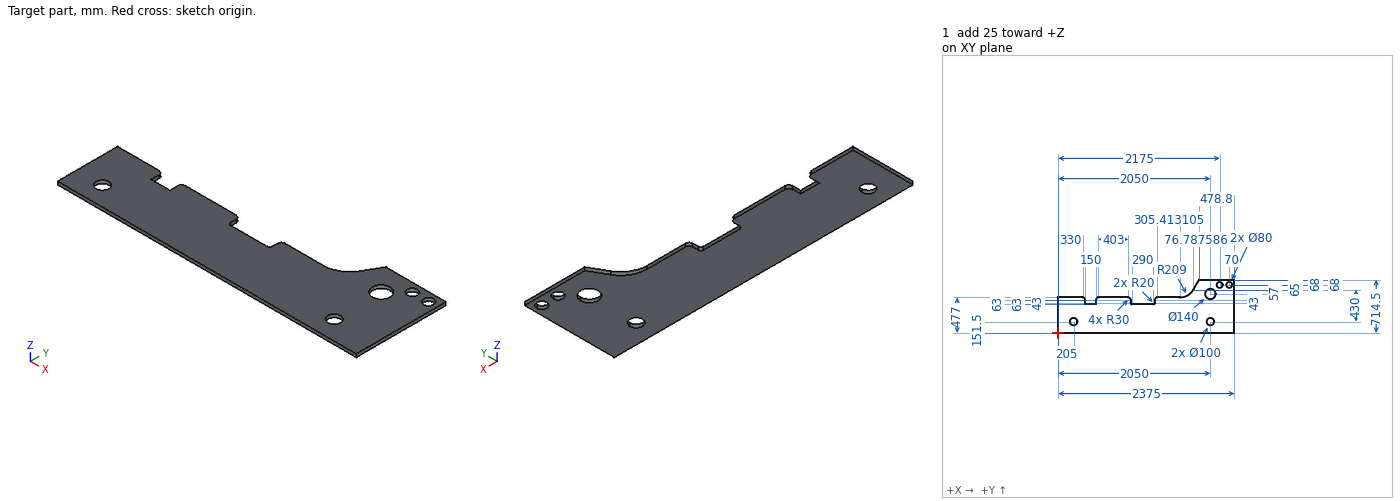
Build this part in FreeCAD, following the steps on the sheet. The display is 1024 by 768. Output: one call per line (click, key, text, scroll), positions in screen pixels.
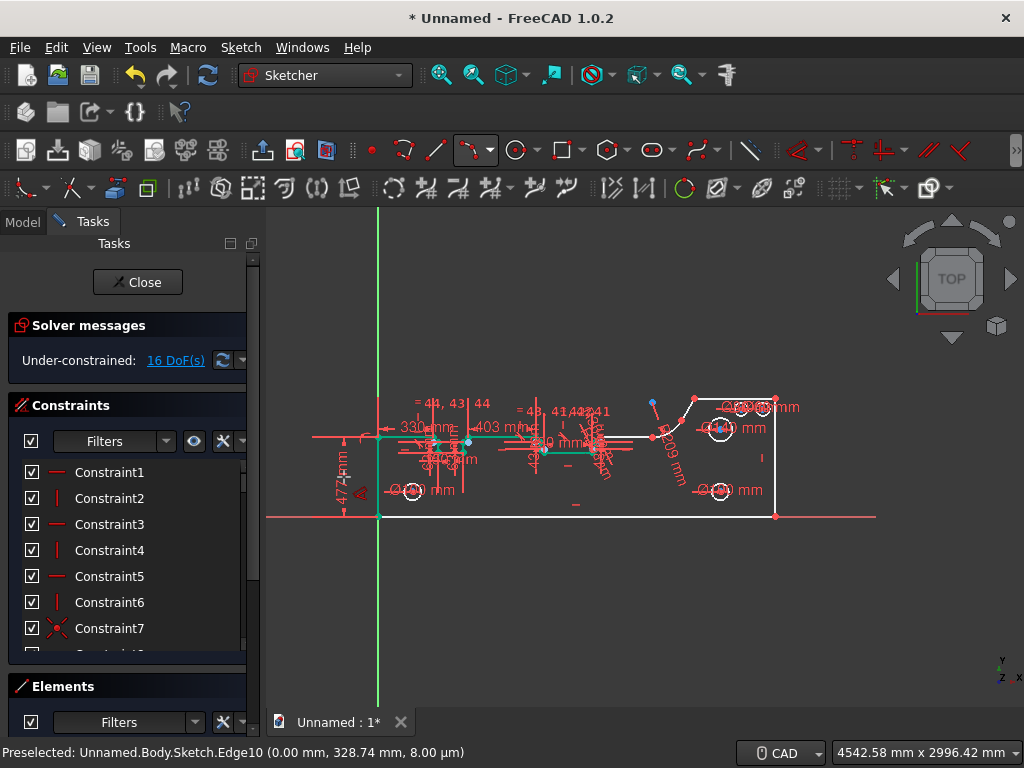
click(413, 492)
click(395, 551)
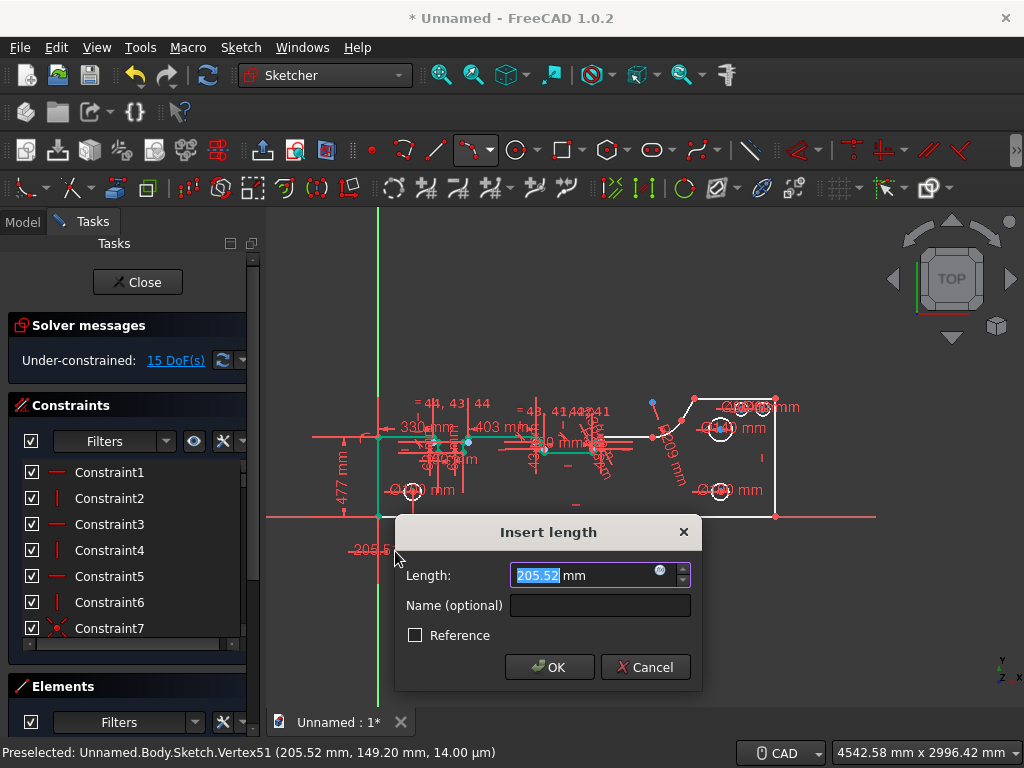
text(205)
key(Return)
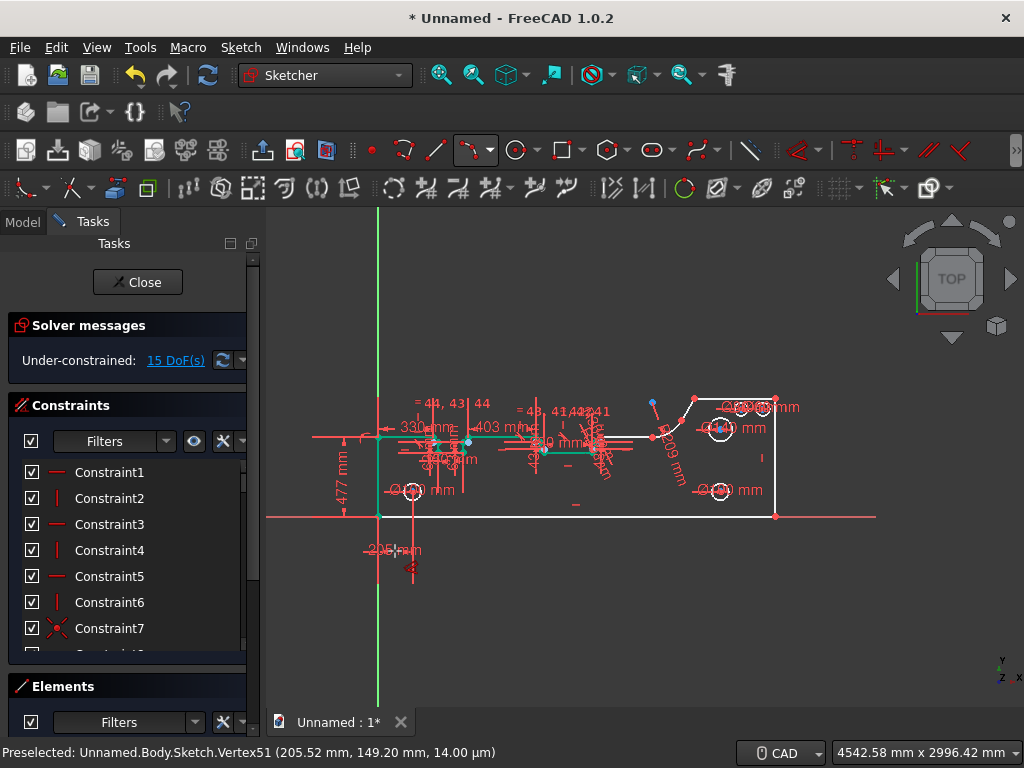
scroll(682, 421, up, 8)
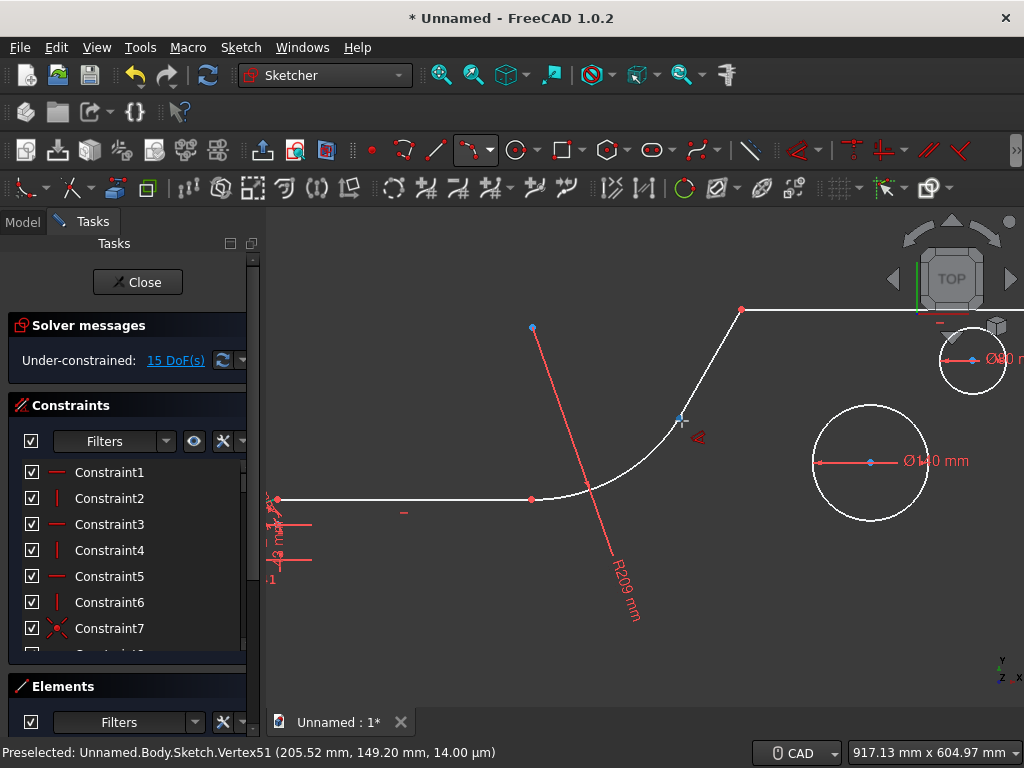
click(679, 418)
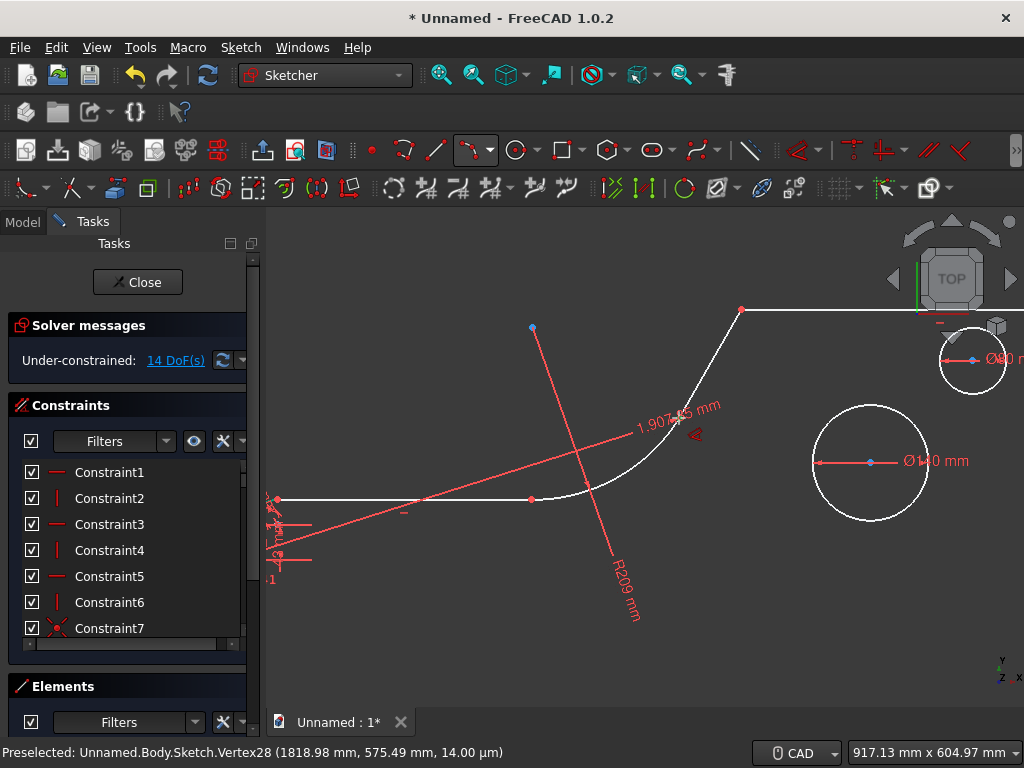
scroll(683, 421, down, 8)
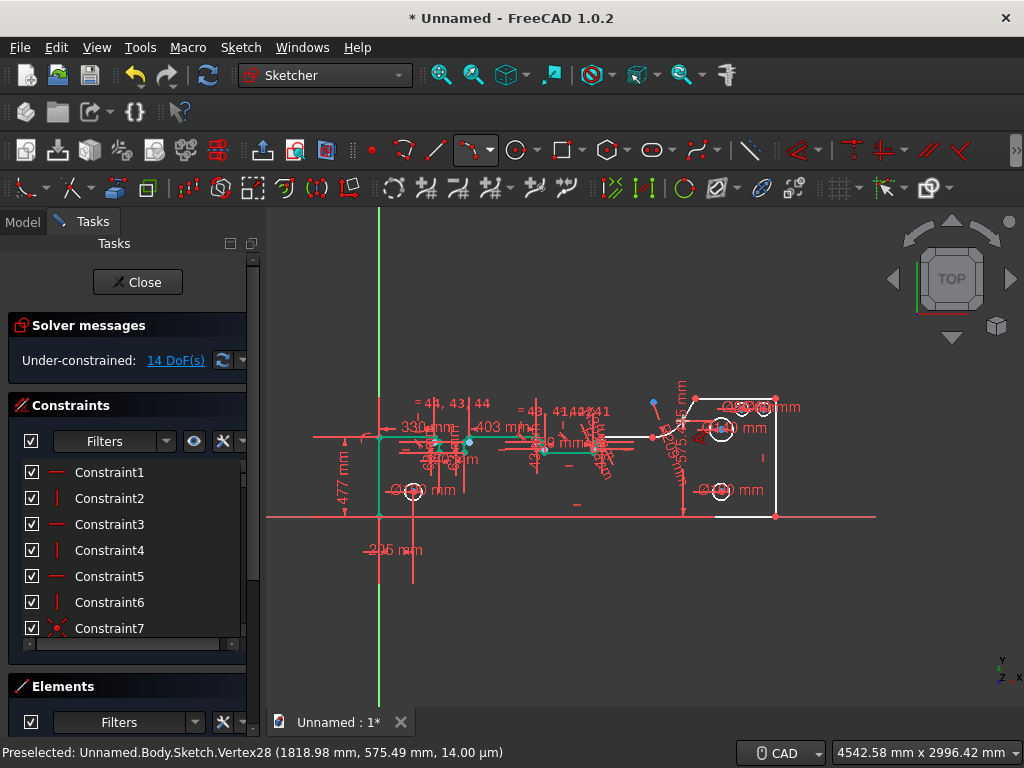
scroll(721, 430, up, 8)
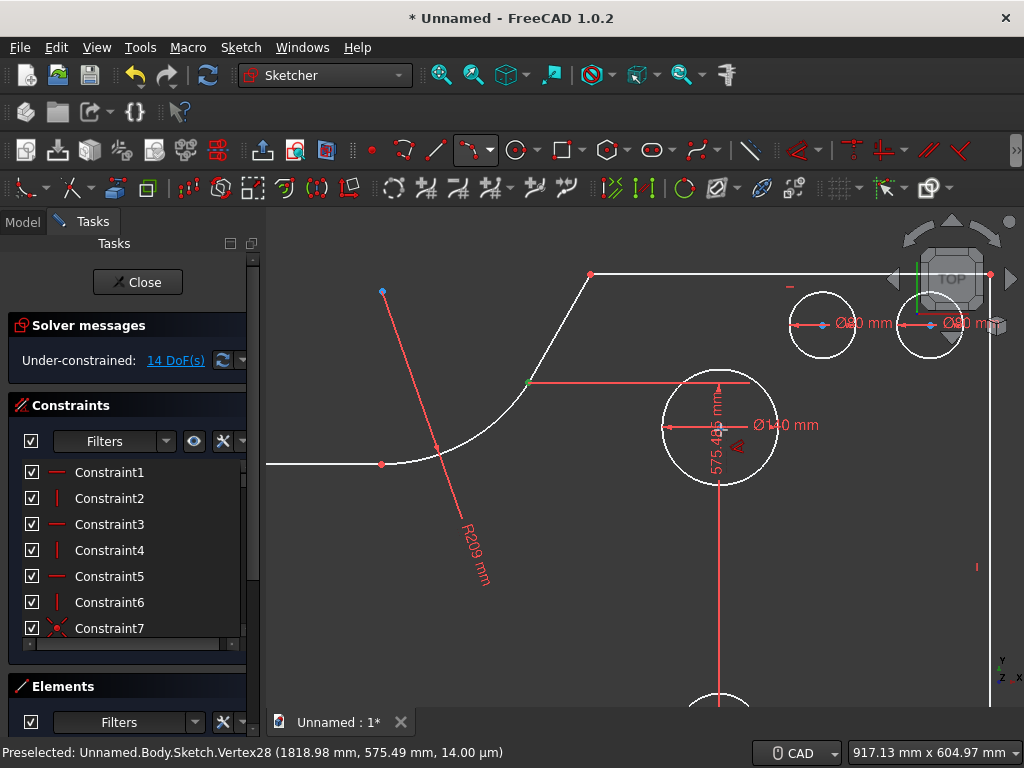
click(720, 427)
click(754, 405)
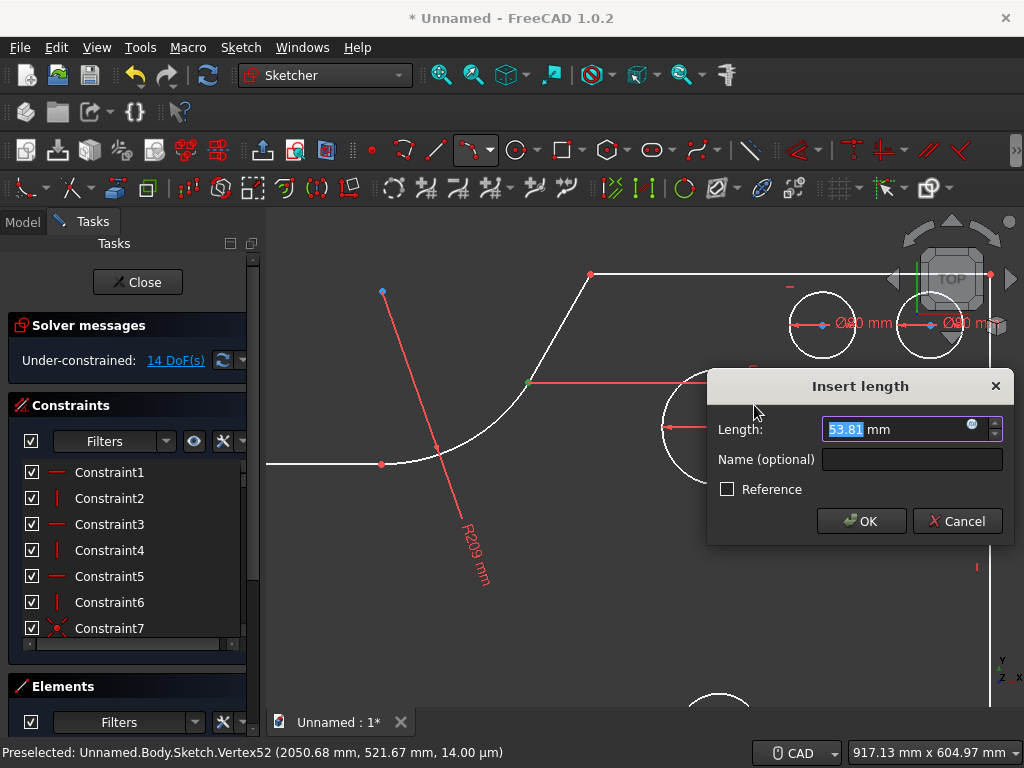
text(57)
key(Return)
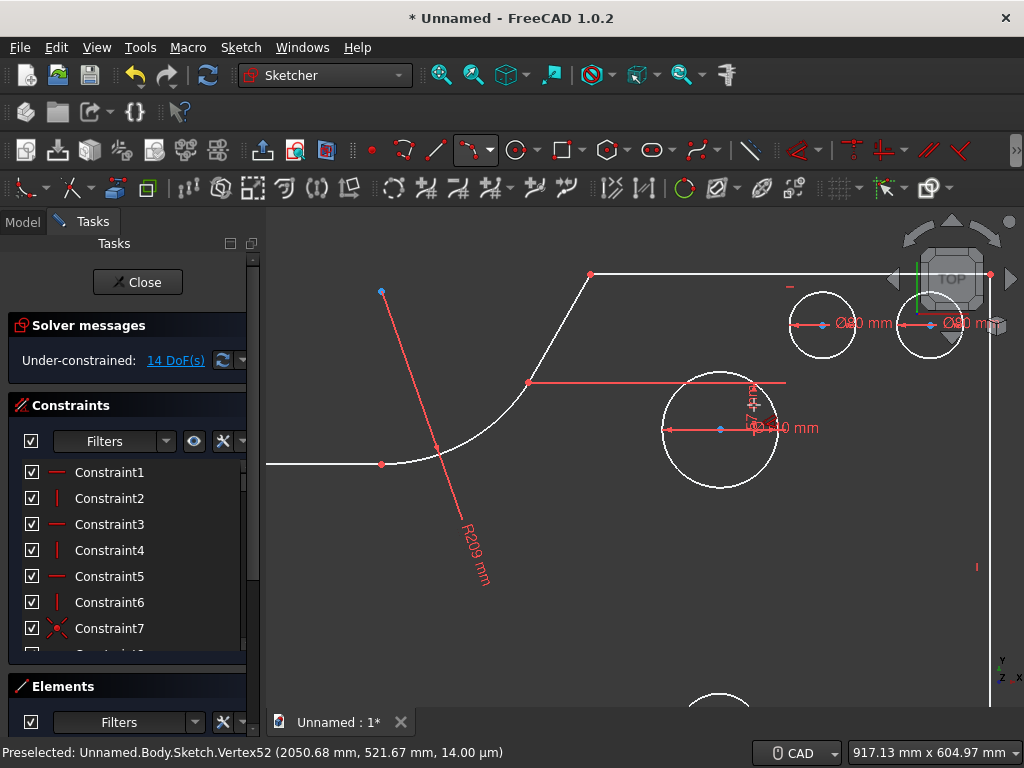
scroll(721, 430, down, 8)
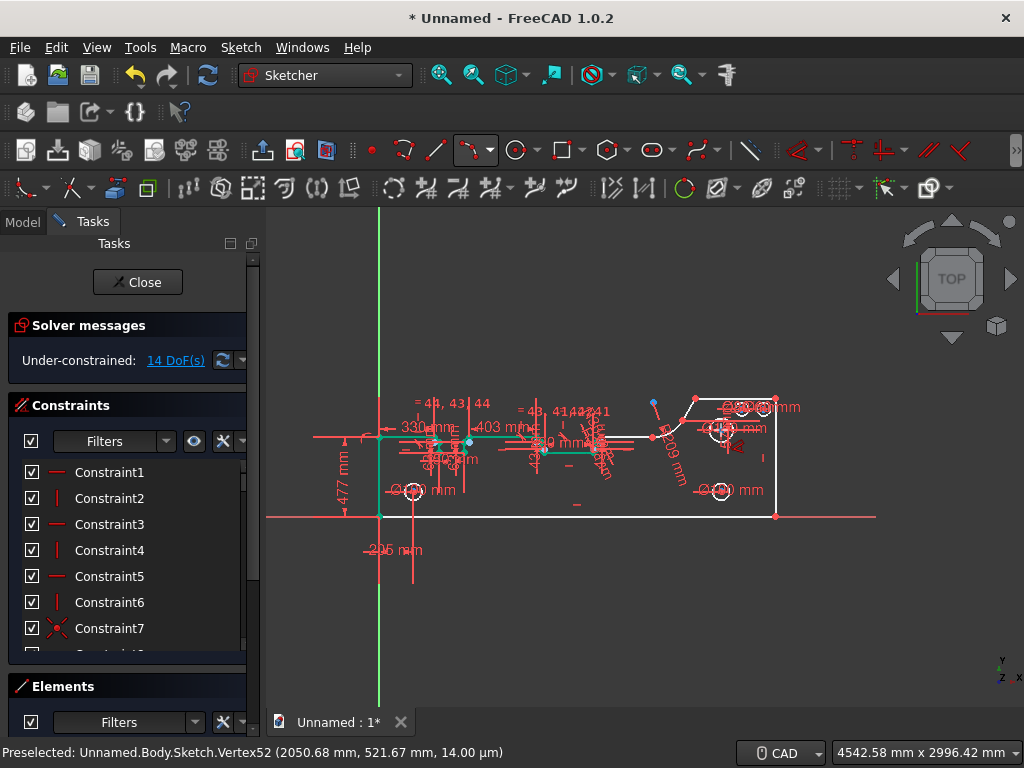
scroll(776, 399, up, 7)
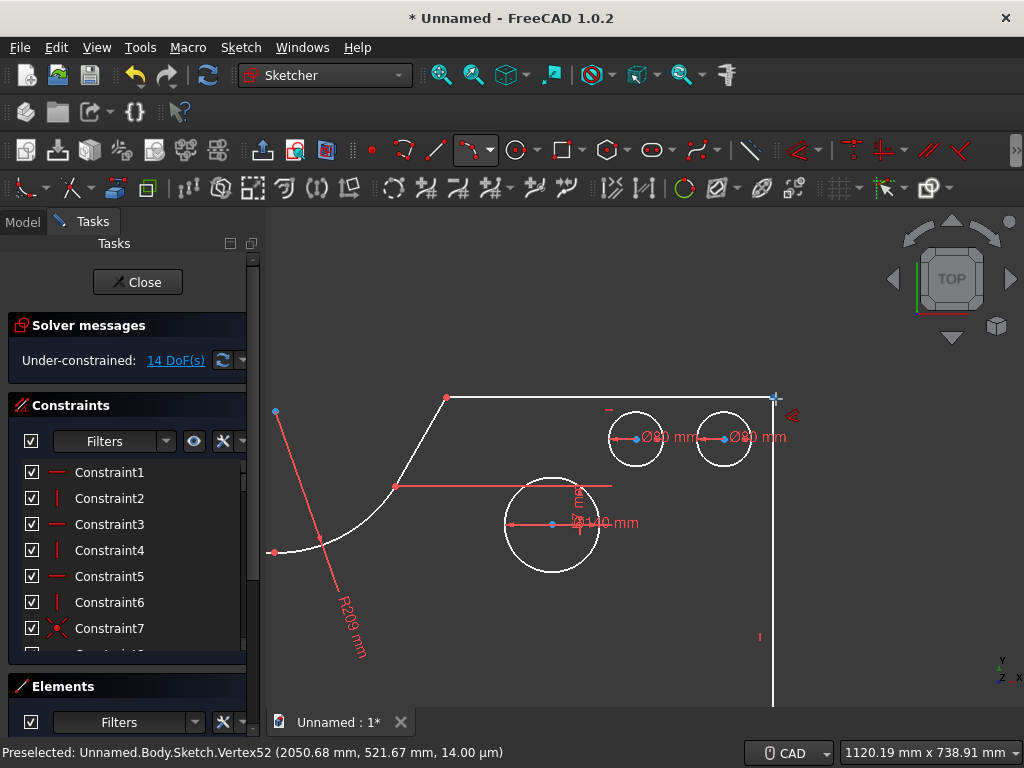
click(773, 397)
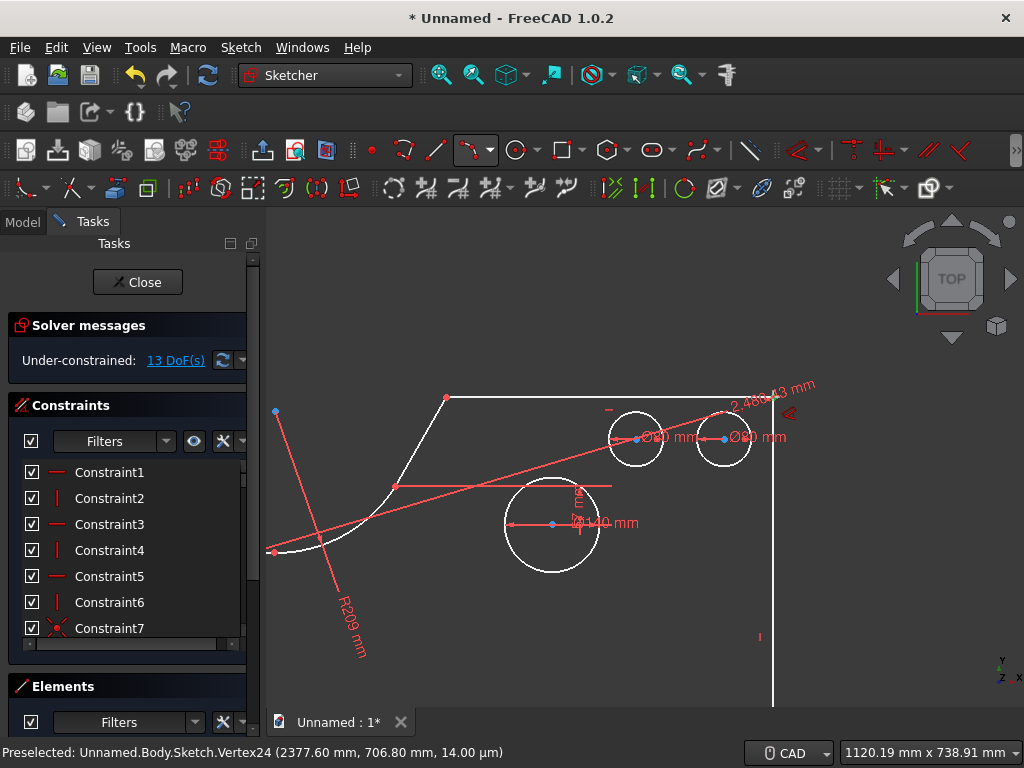
click(724, 439)
click(749, 363)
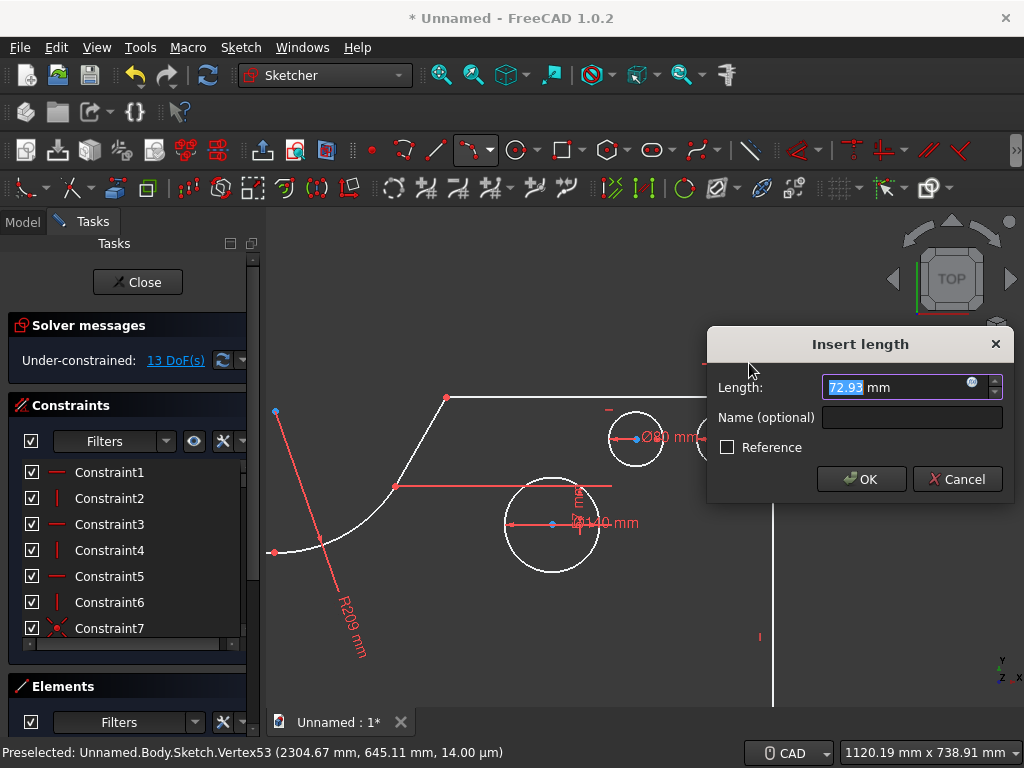
text(70)
key(Return)